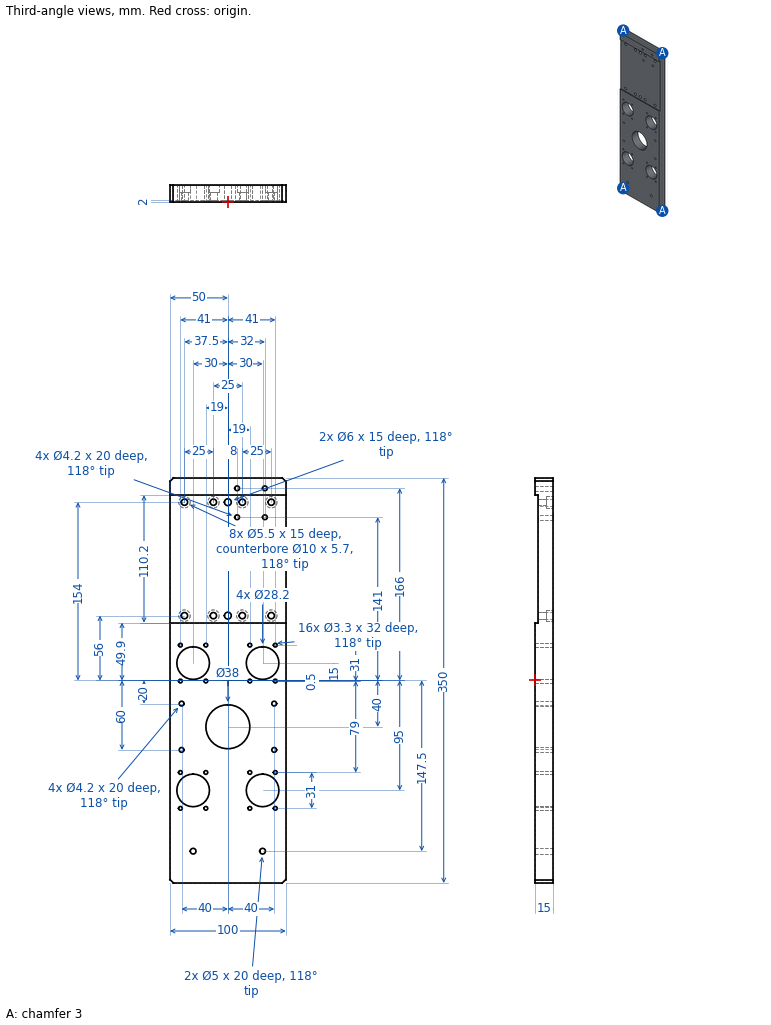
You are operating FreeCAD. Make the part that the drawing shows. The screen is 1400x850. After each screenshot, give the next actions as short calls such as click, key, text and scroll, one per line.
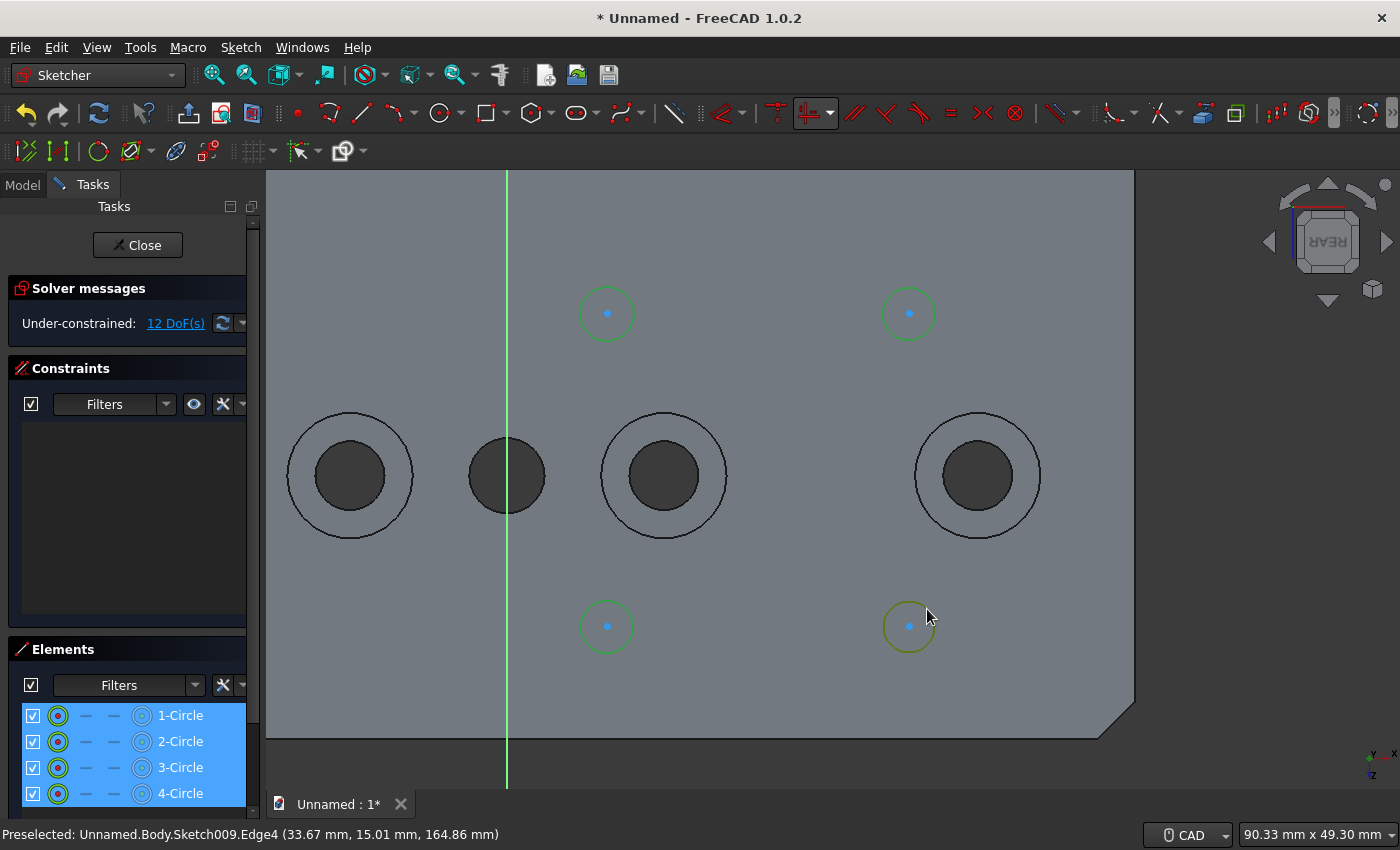
key(e)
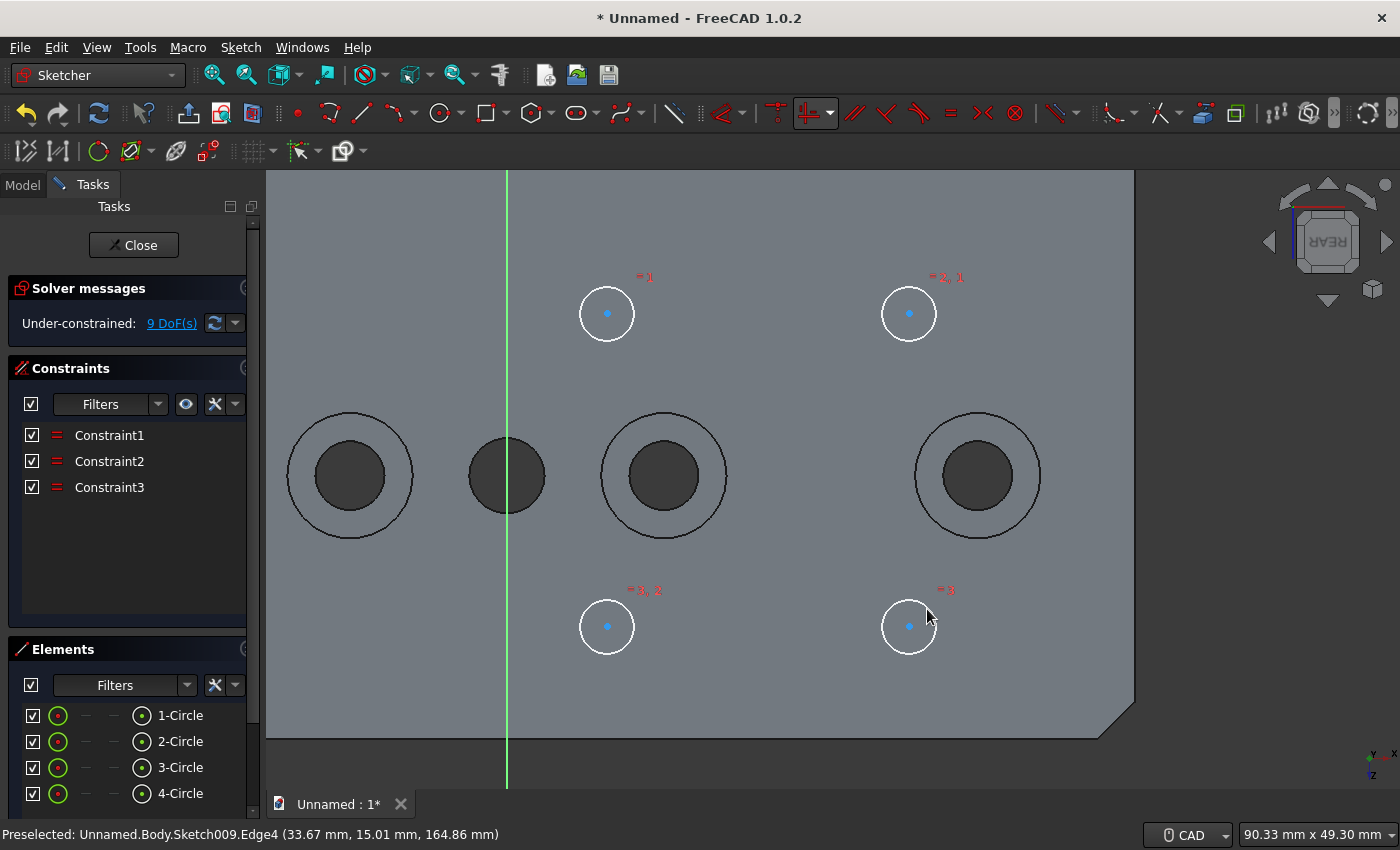
click(607, 314)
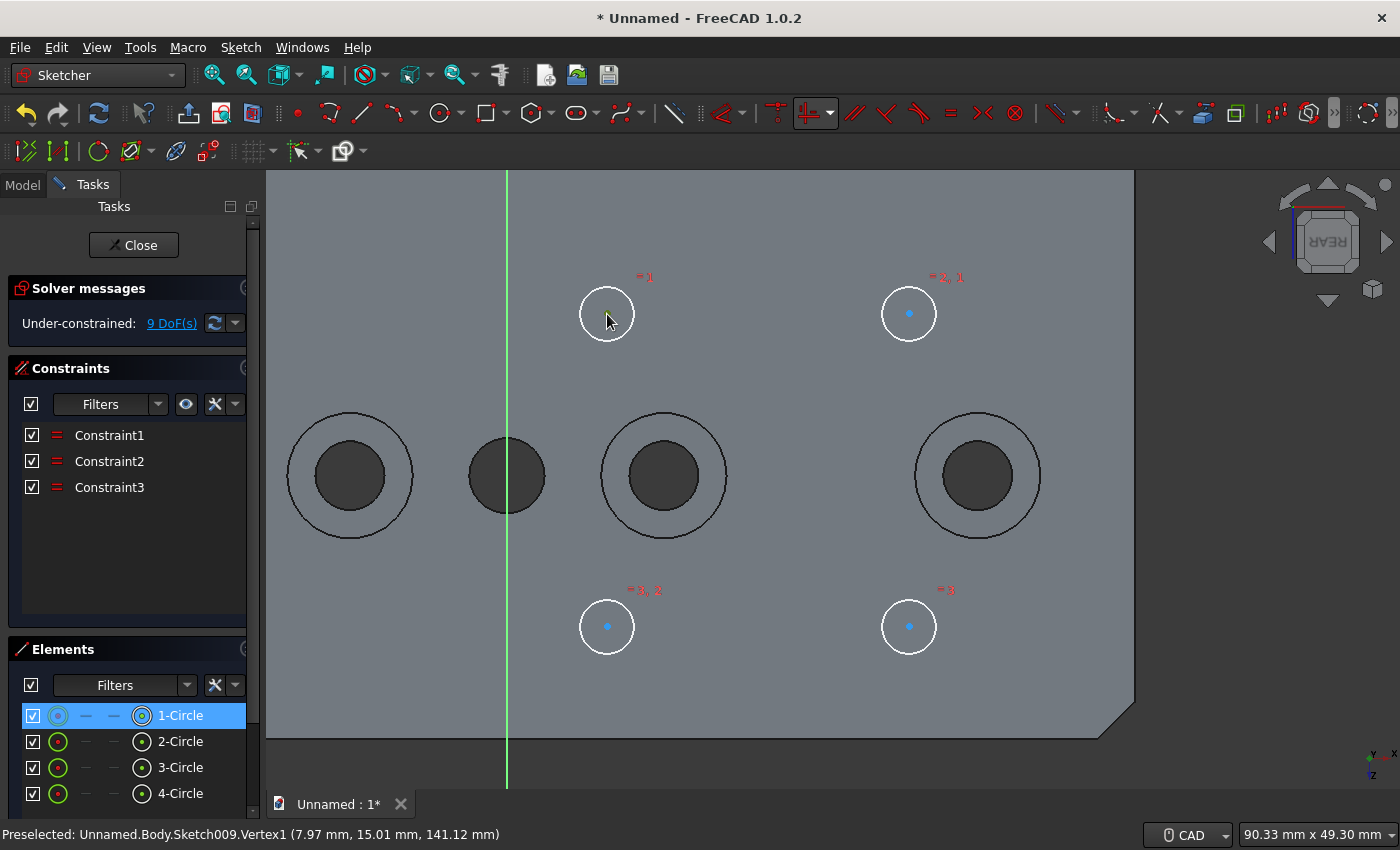
click(909, 314)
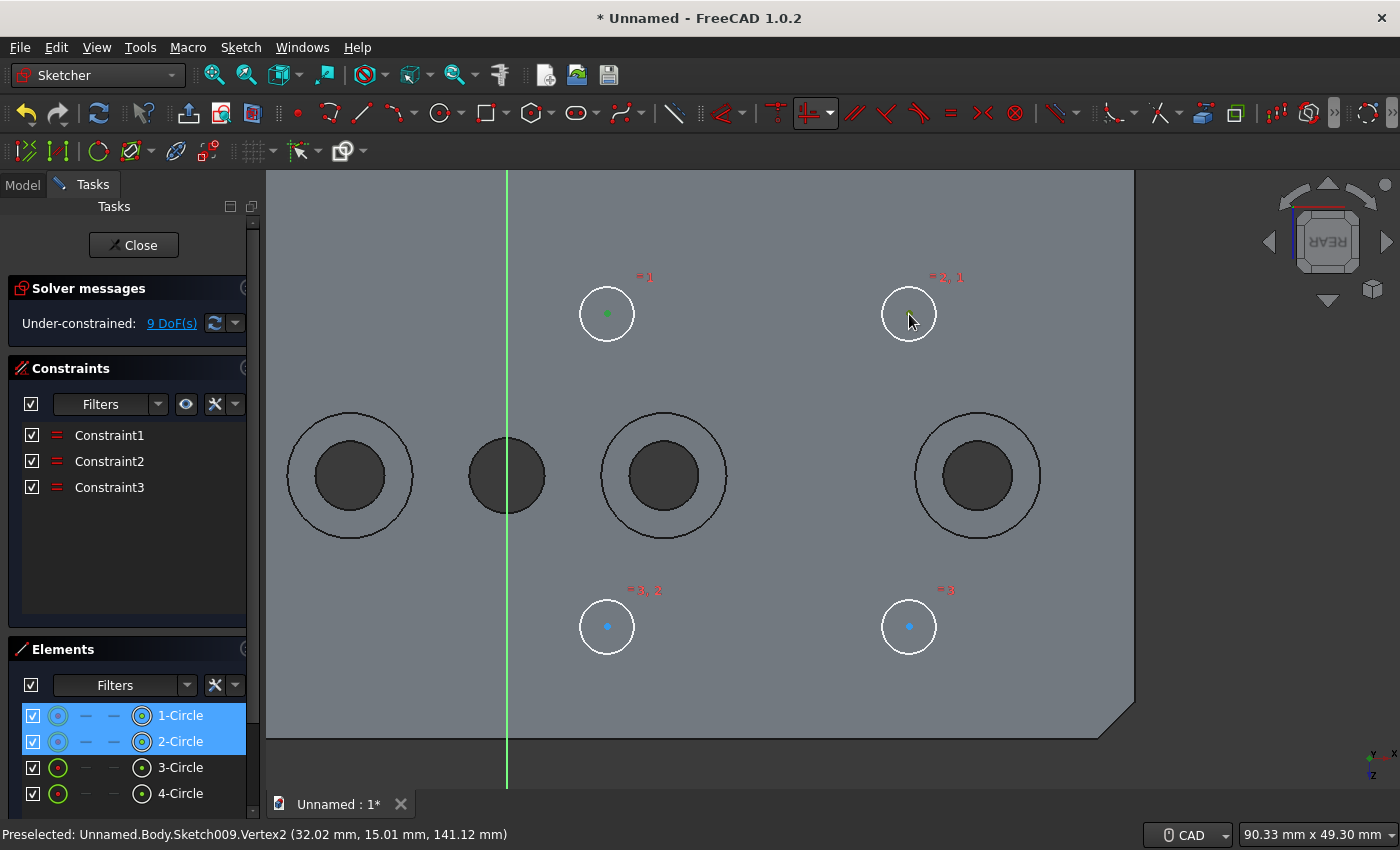
key(h)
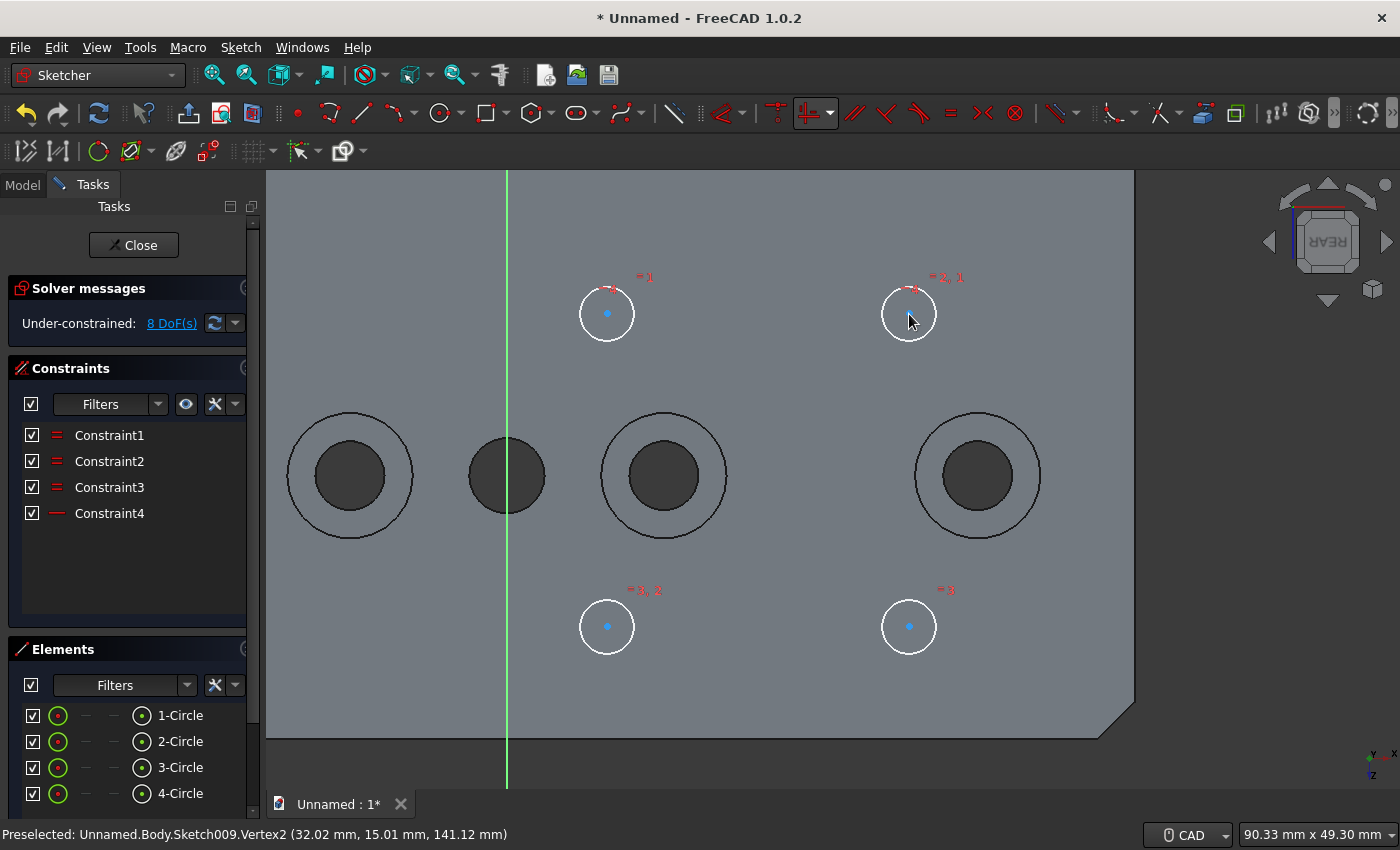
click(607, 314)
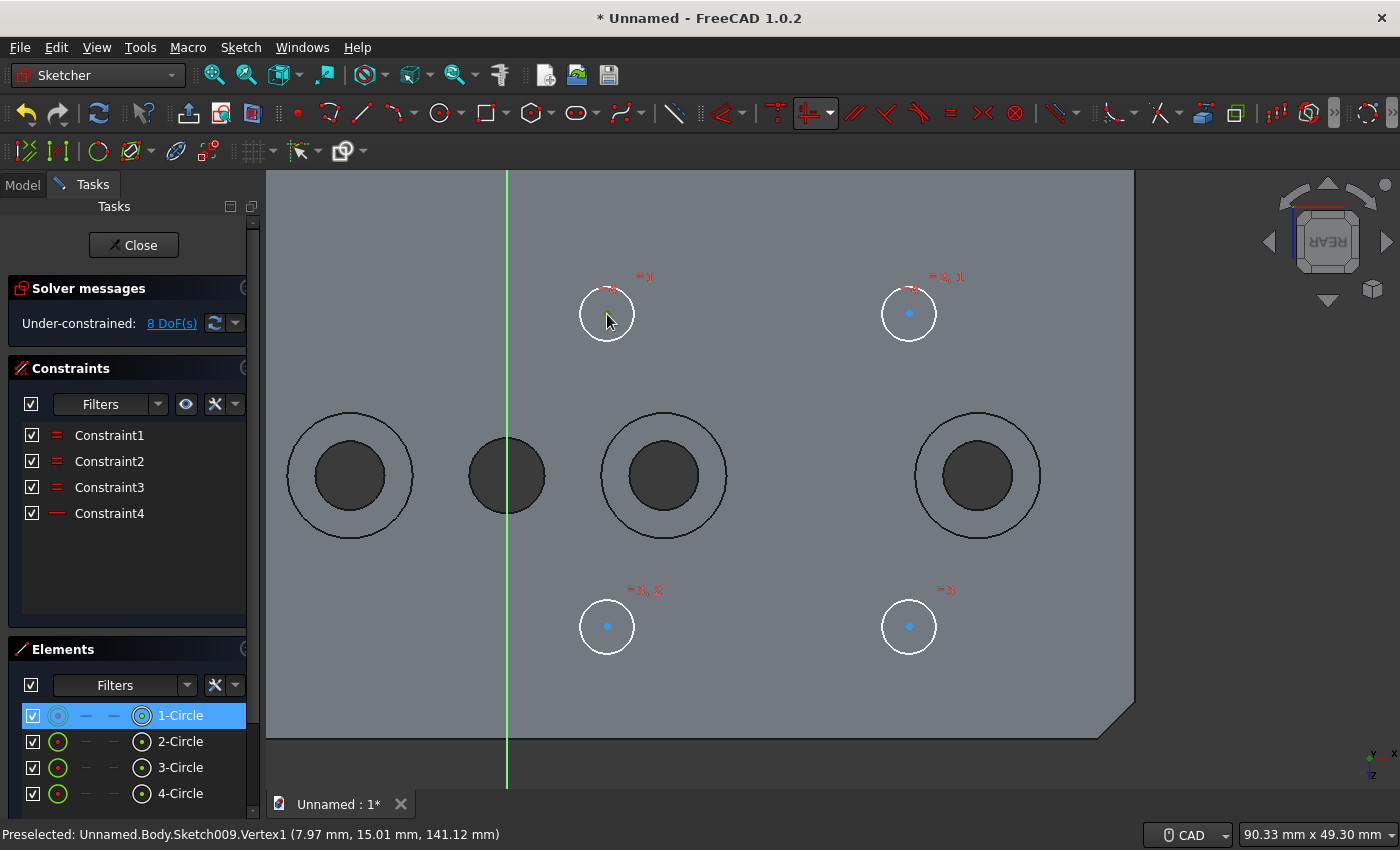
click(607, 627)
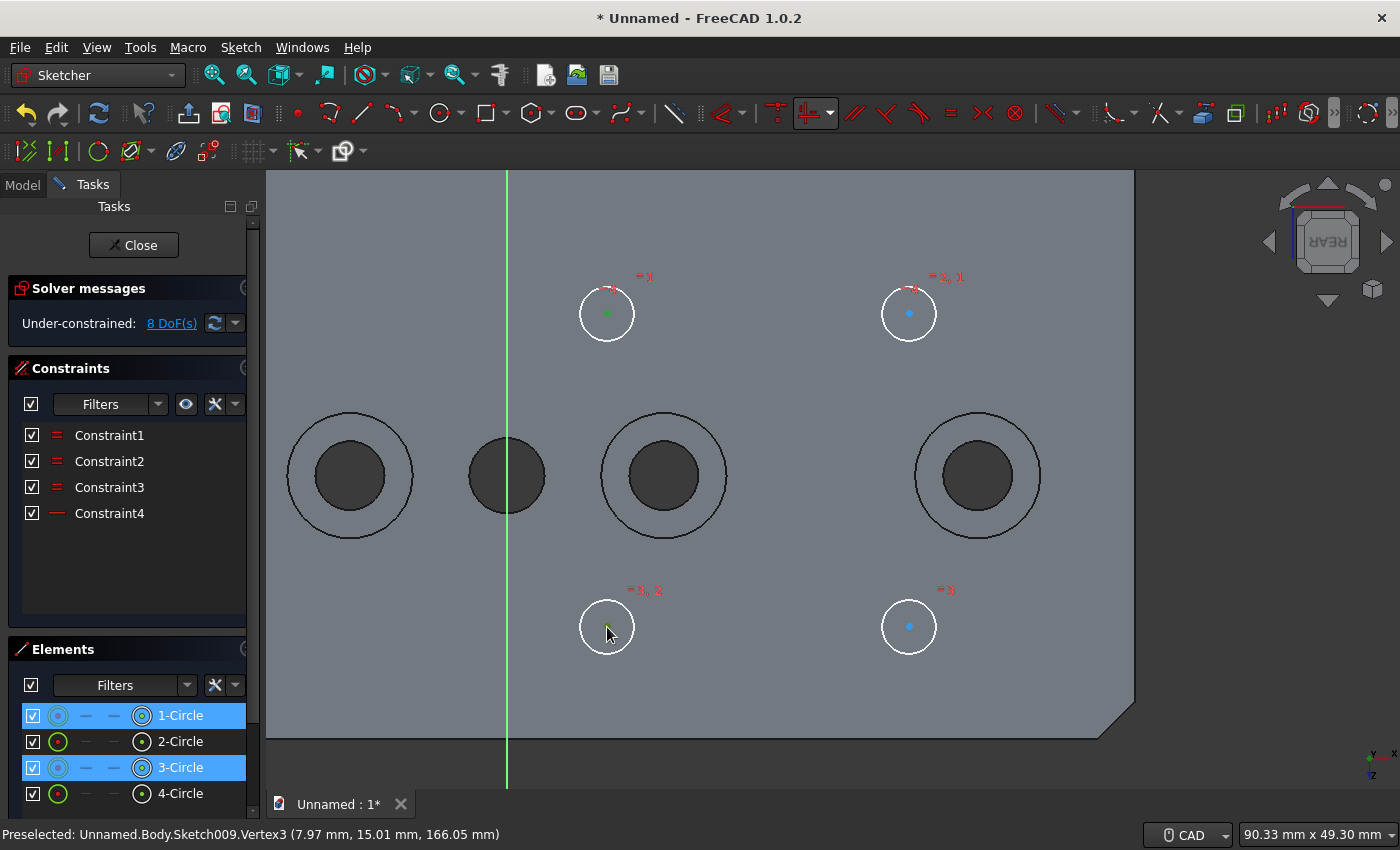
click(832, 114)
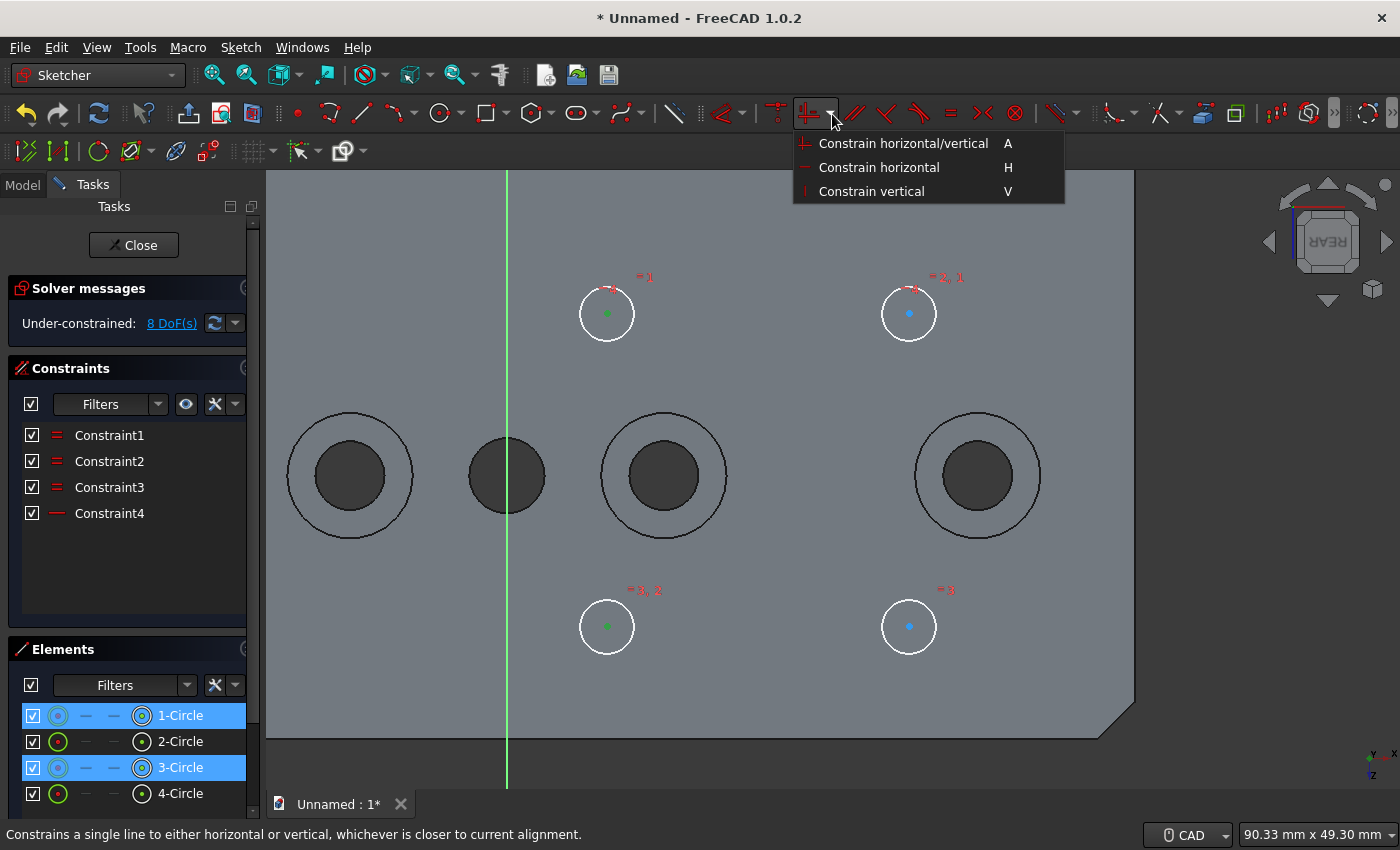
click(929, 191)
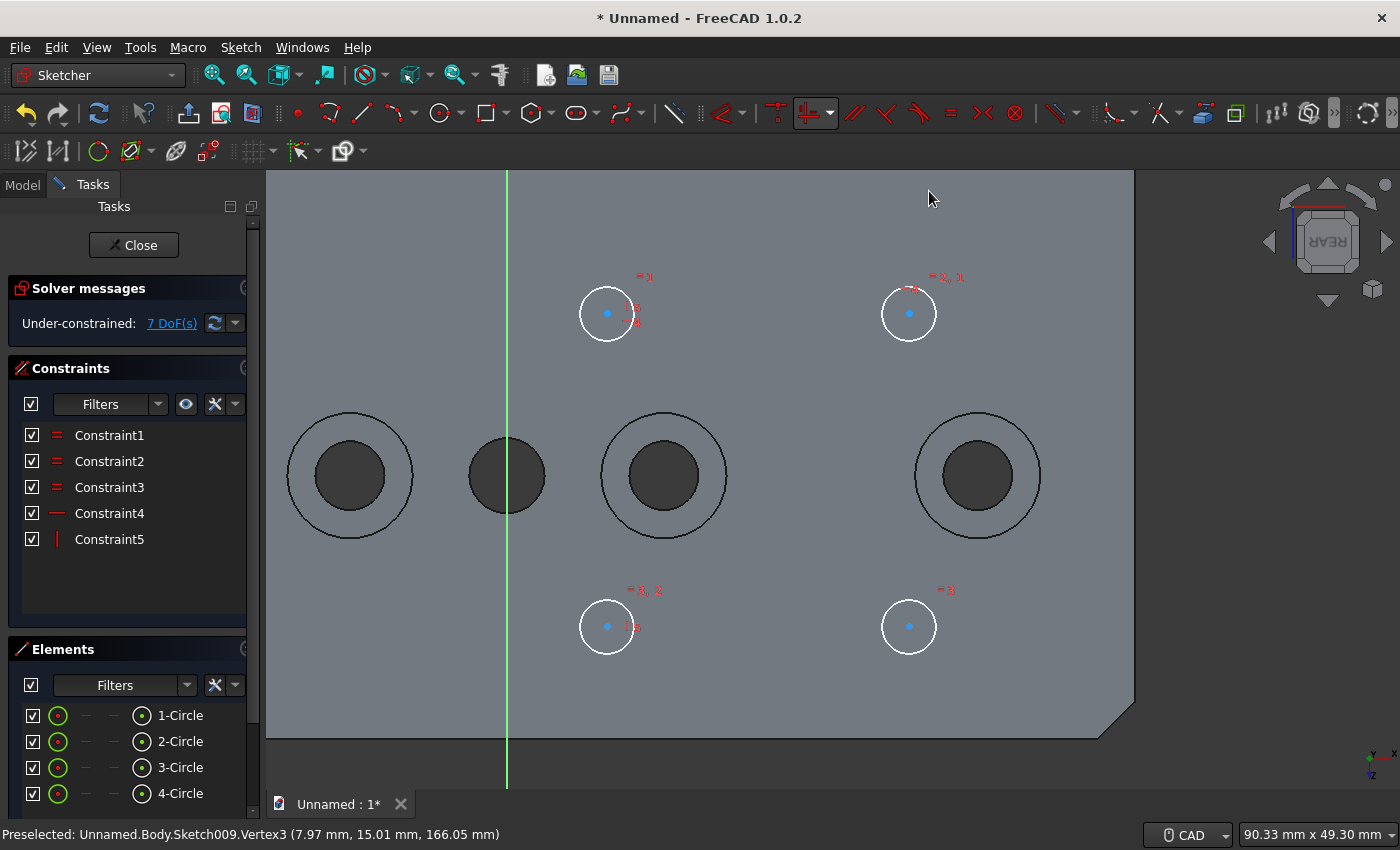
click(909, 314)